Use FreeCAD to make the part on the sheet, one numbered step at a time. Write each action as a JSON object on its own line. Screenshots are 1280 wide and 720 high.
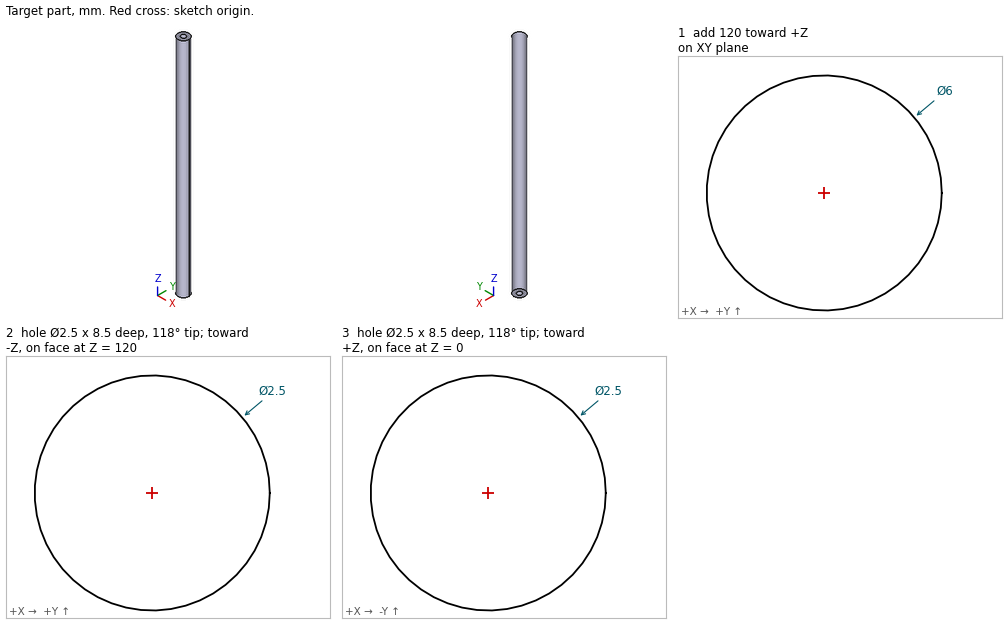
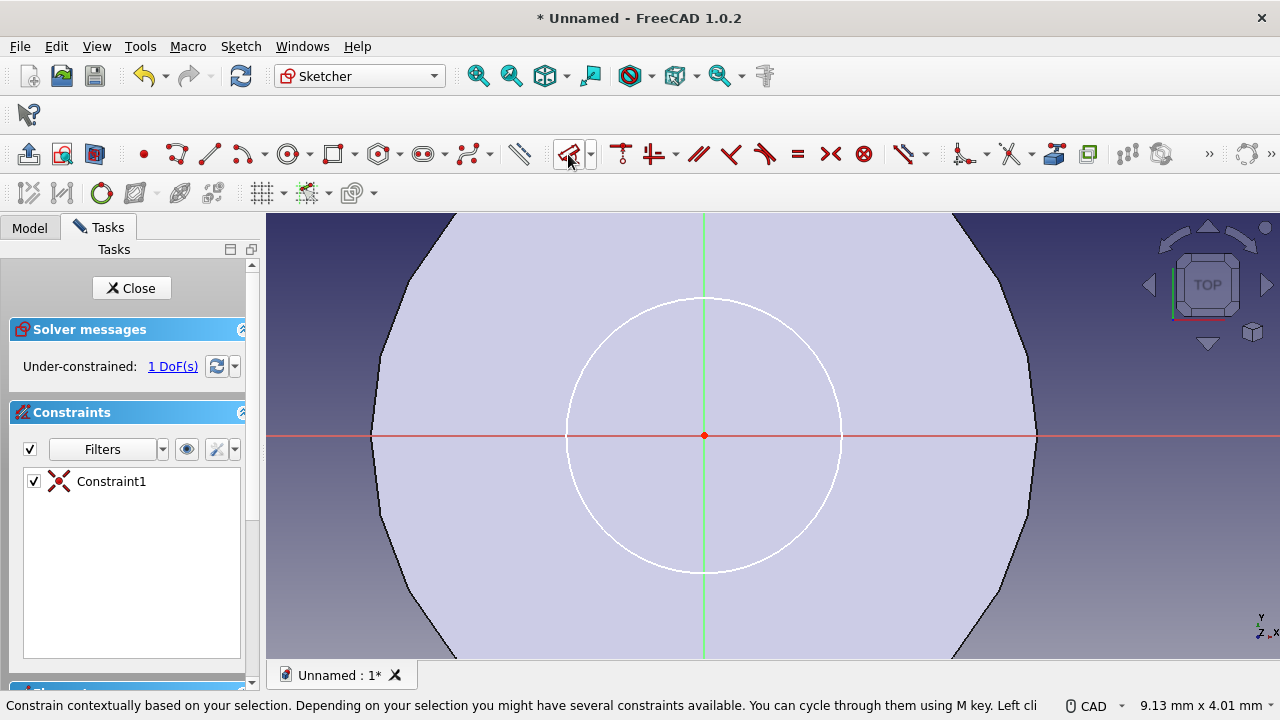
{"action": "left_click", "coordinate": [801, 338]}
{"action": "left_click", "coordinate": [824, 315]}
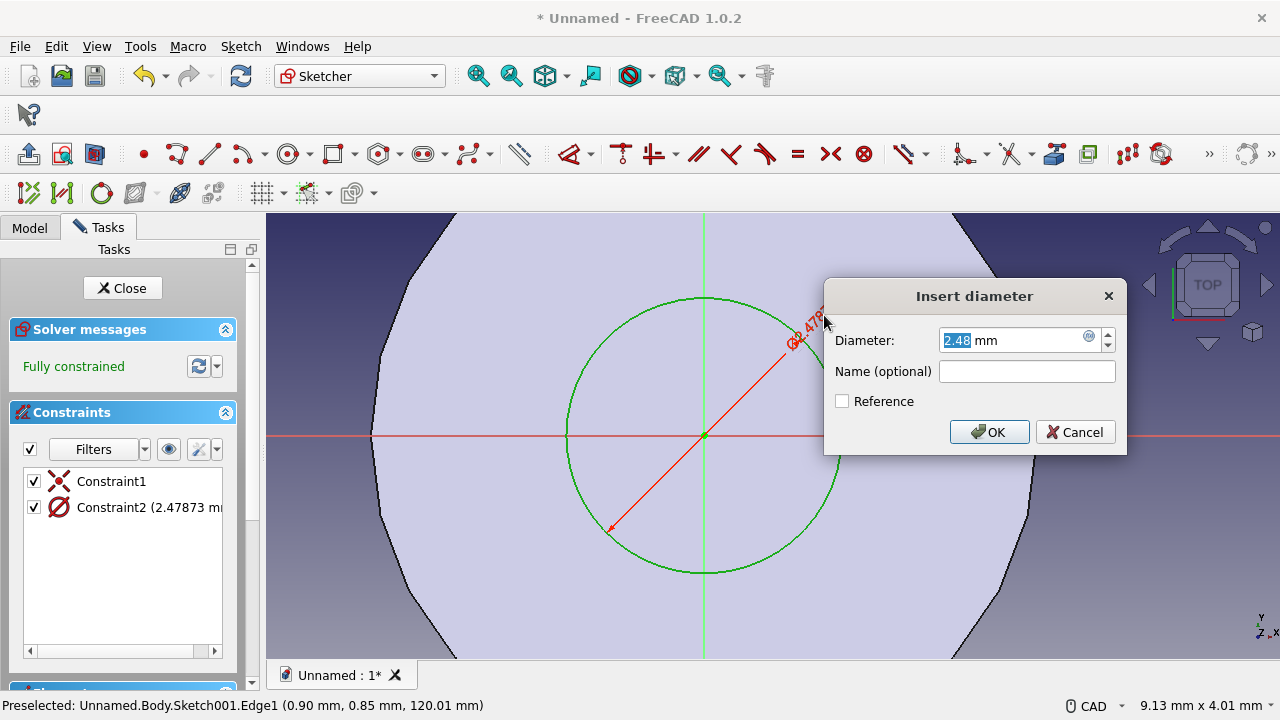
{"action": "type", "text": "2.5"}
{"action": "key", "text": "Return"}
{"action": "key", "text": "Escape"}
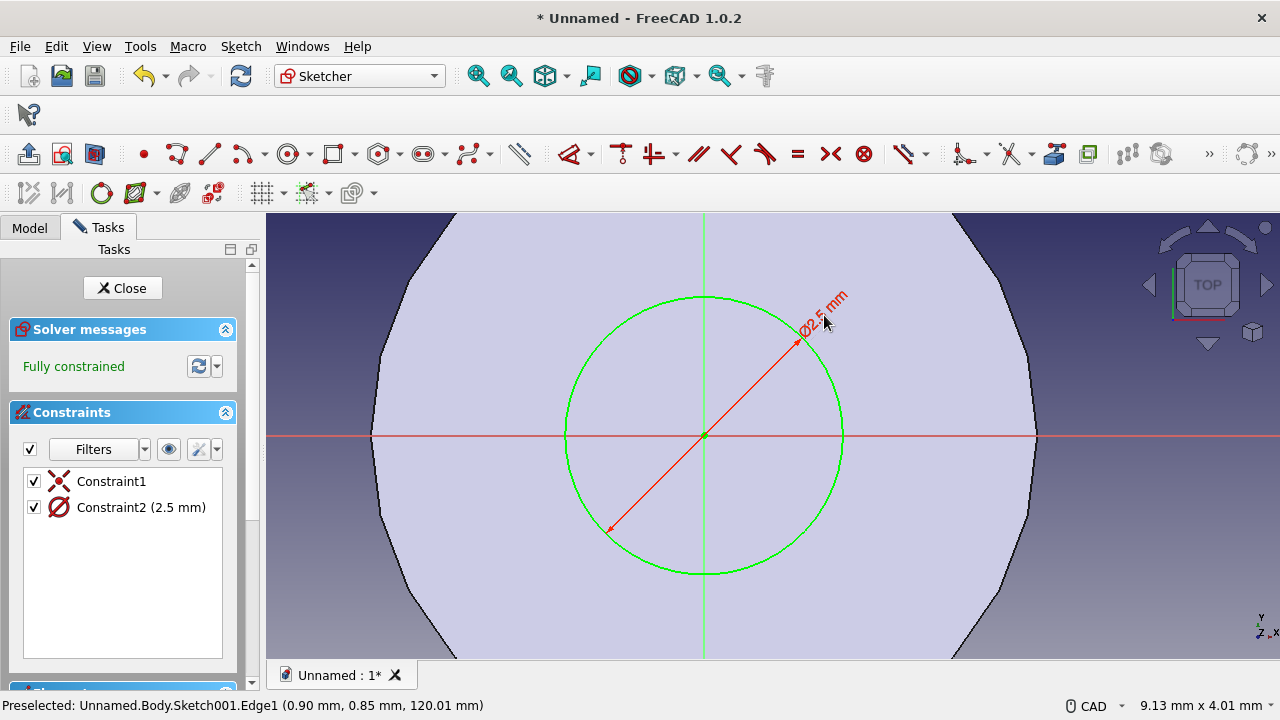
{"action": "left_click", "coordinate": [123, 288]}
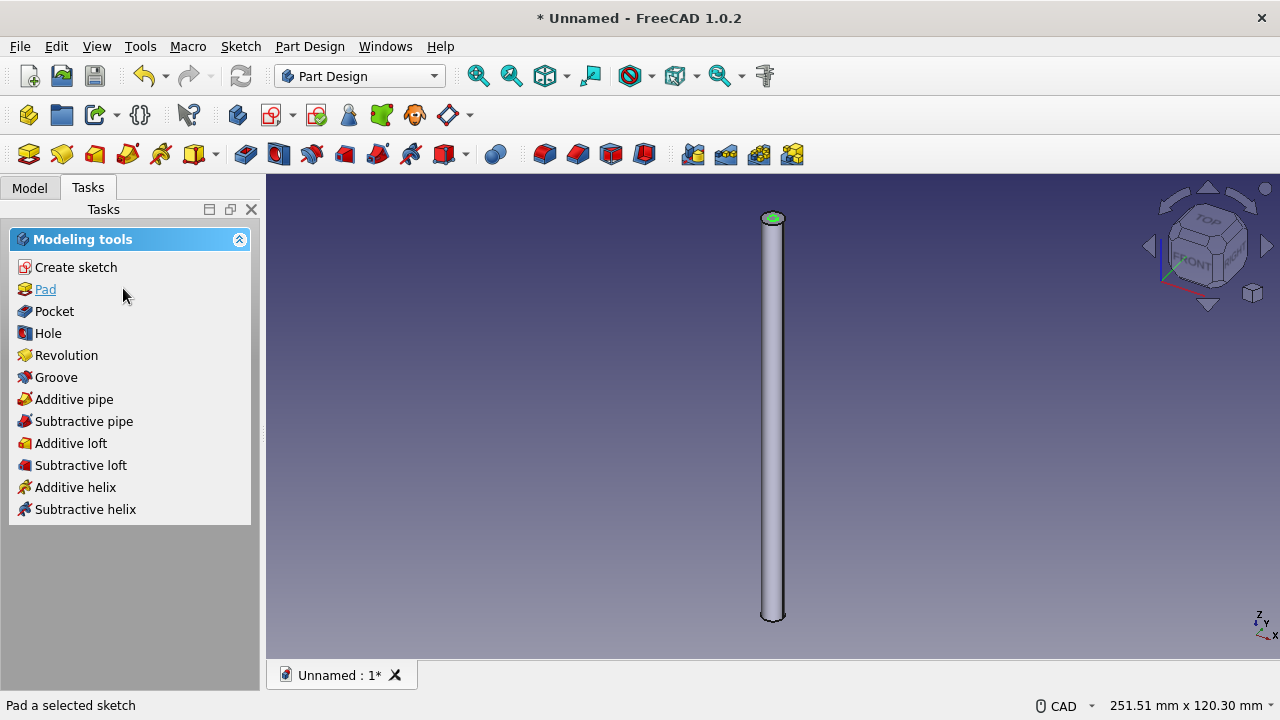
{"action": "left_click", "coordinate": [279, 154]}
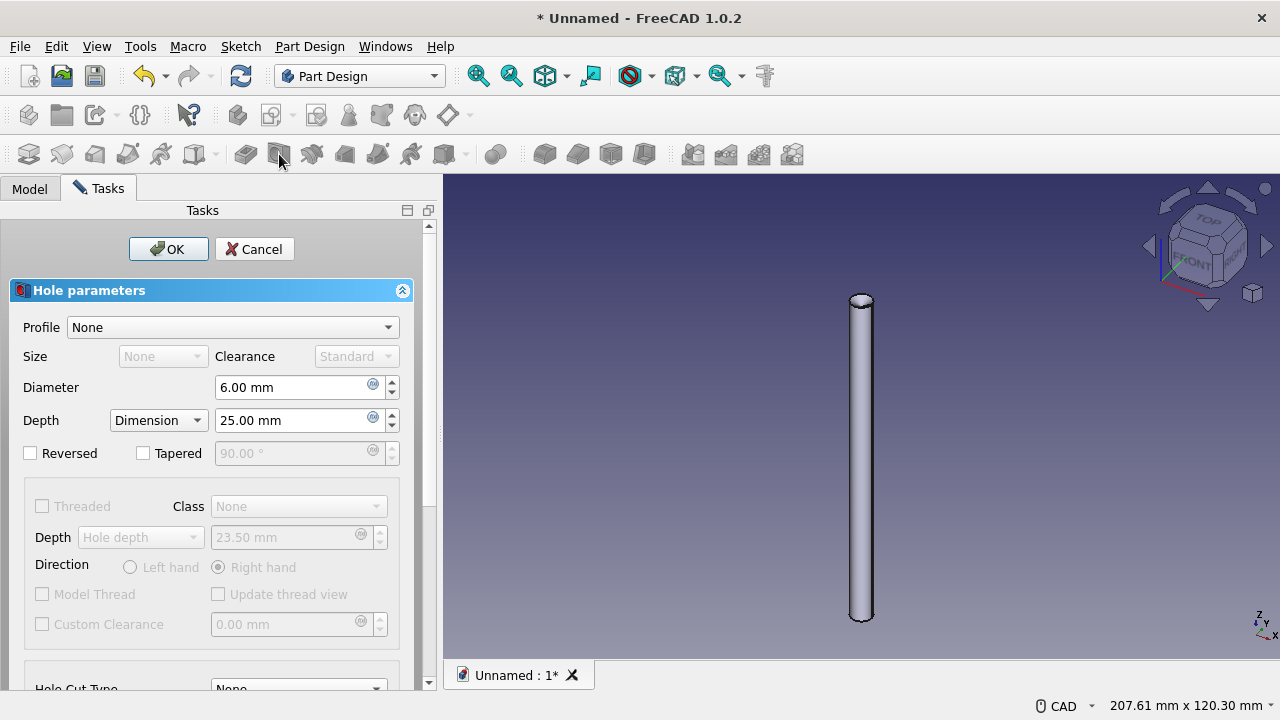
{"action": "triple_click", "coordinate": [300, 388]}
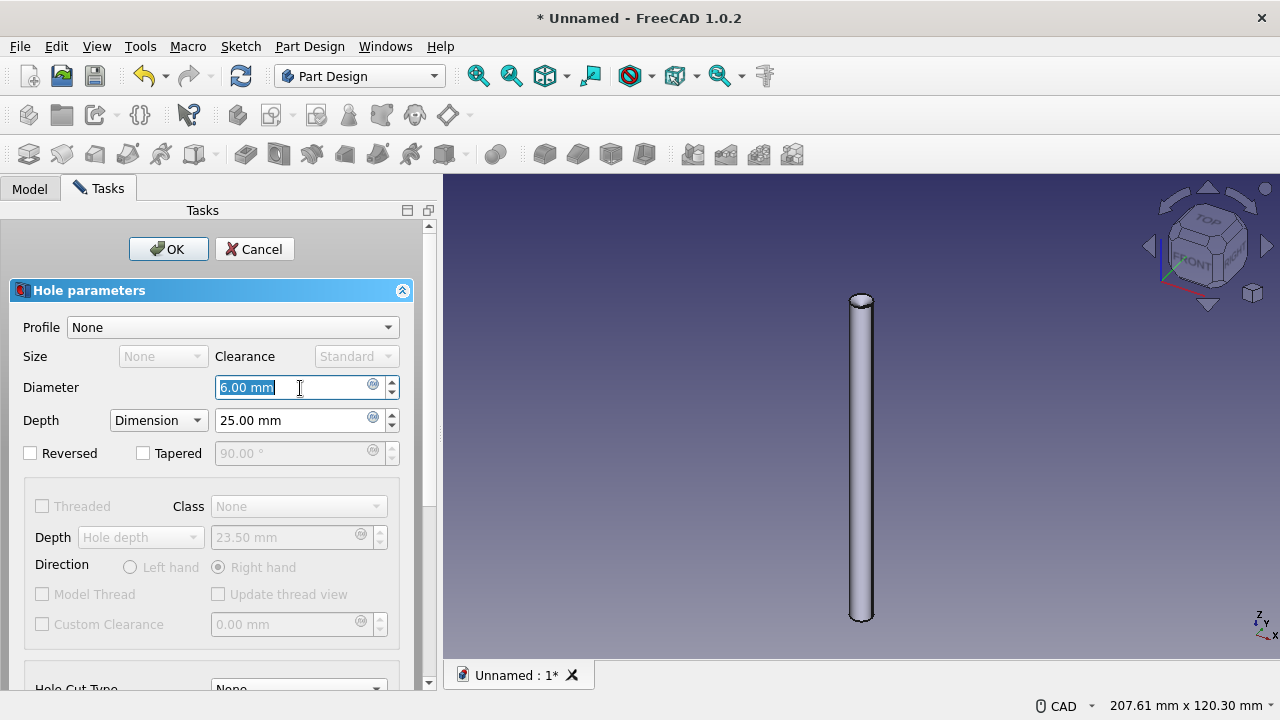
{"action": "type", "text": "2.5"}
{"action": "key", "text": "Tab"}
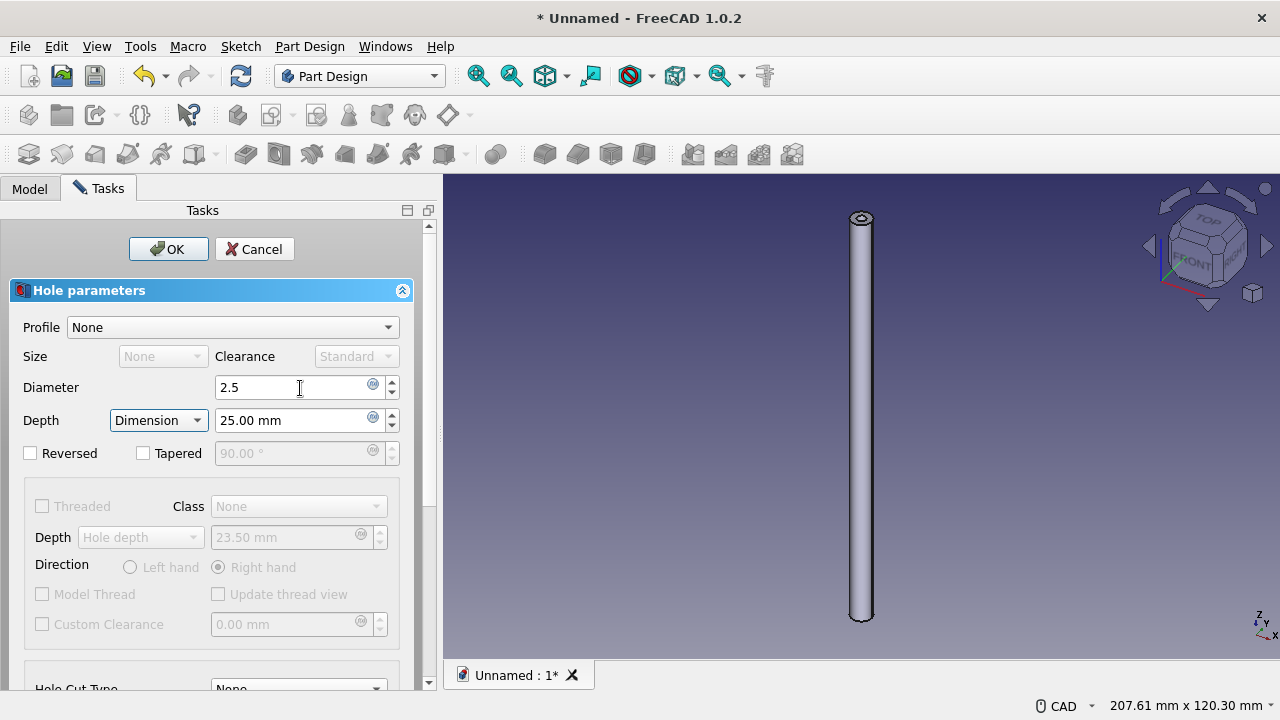
{"action": "triple_click", "coordinate": [300, 420]}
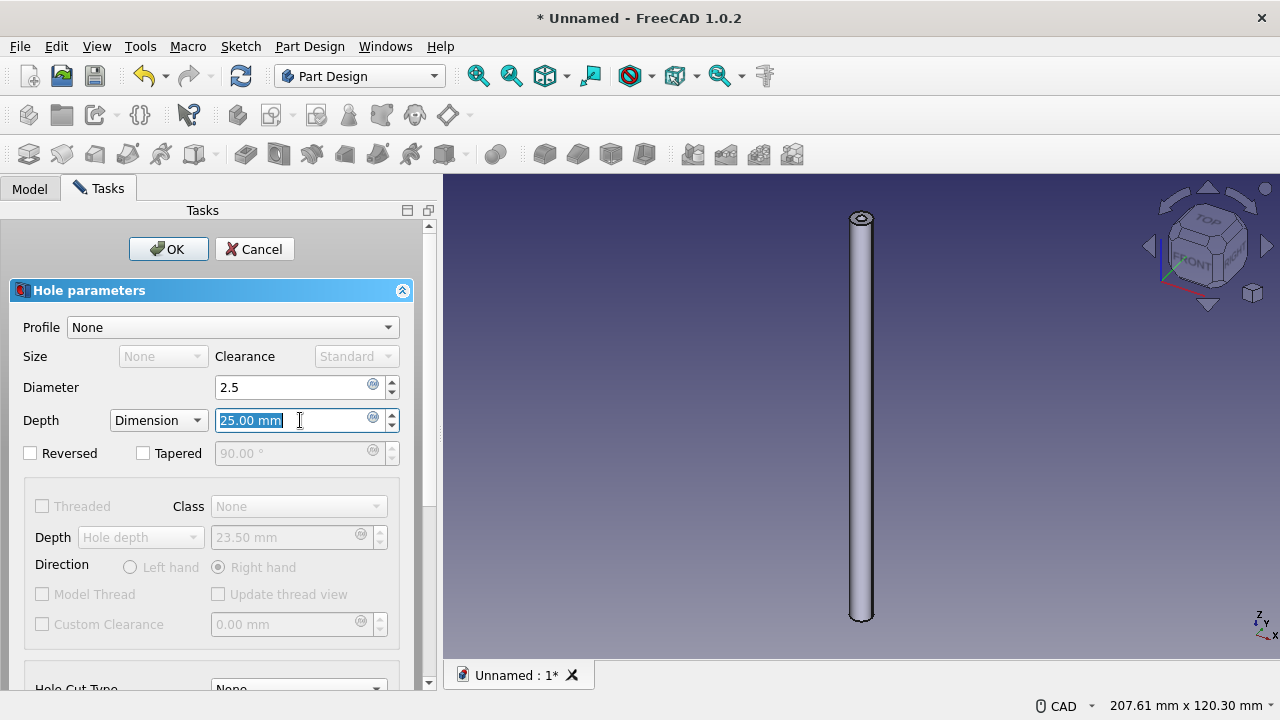
{"action": "type", "text": "8.5"}
{"action": "key", "text": "Tab"}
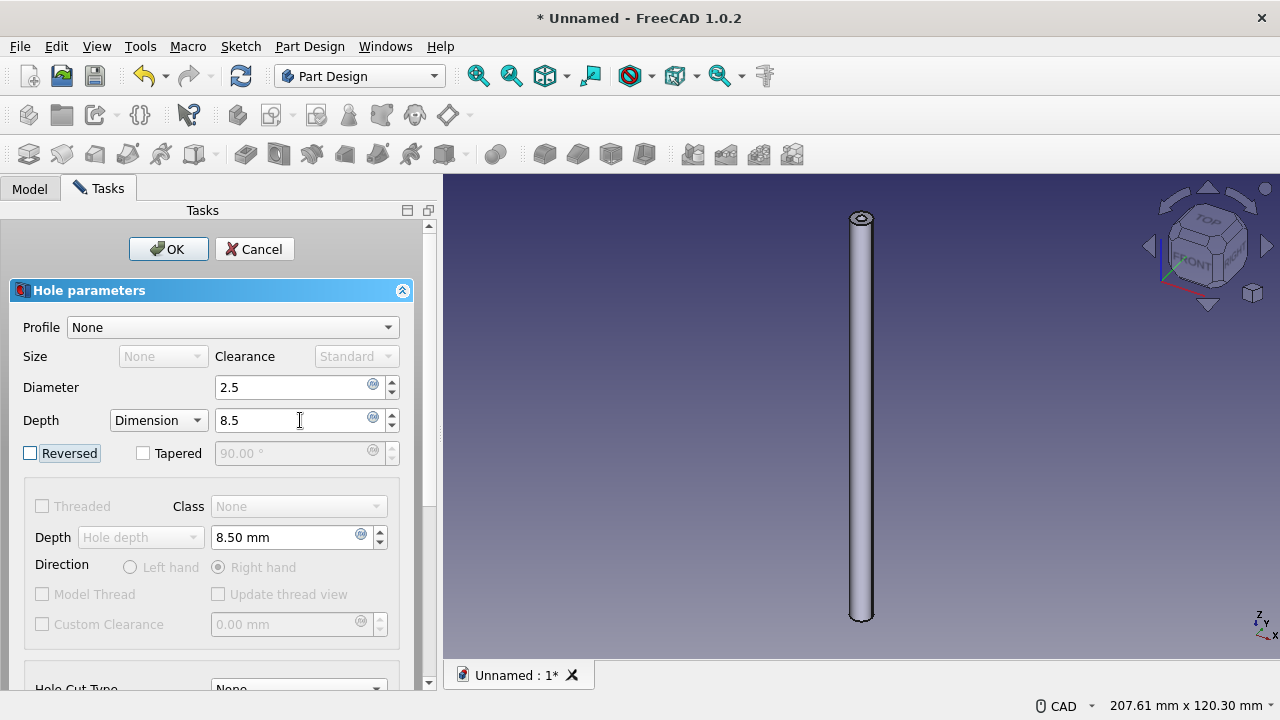
{"action": "left_click", "coordinate": [169, 249]}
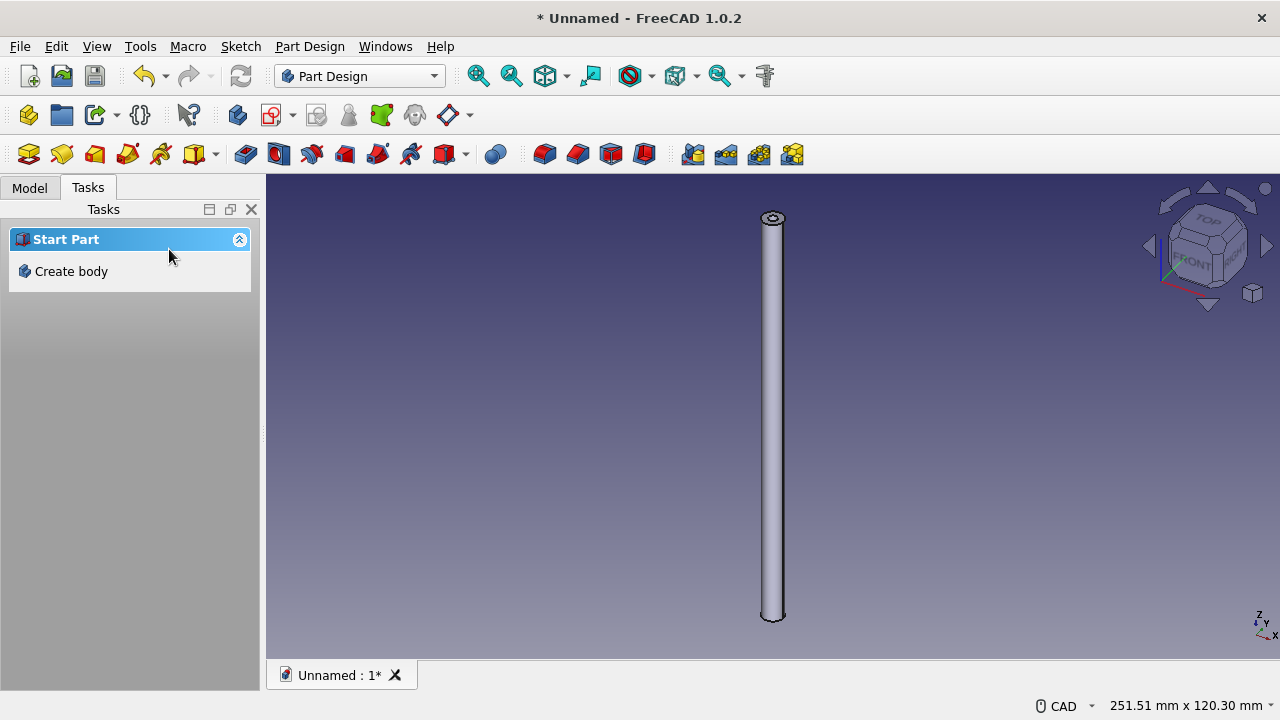
{"action": "key", "text": "5"}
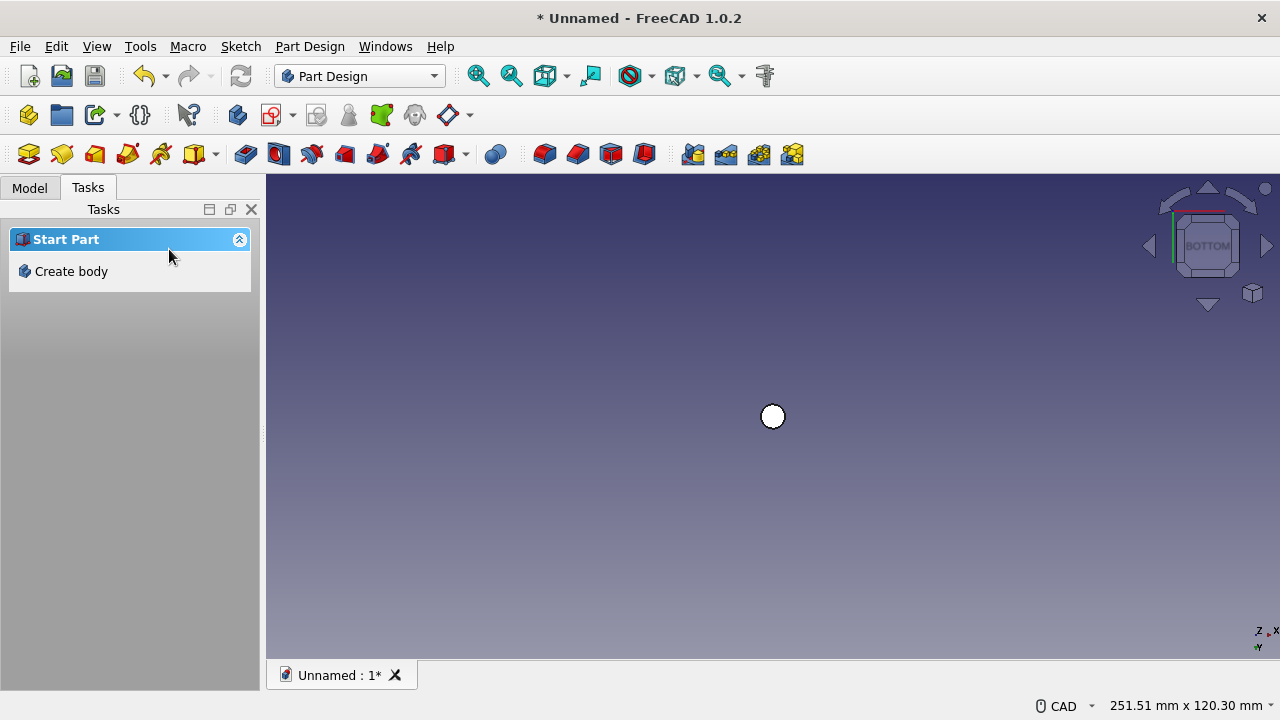
{"action": "key", "text": "v f"}